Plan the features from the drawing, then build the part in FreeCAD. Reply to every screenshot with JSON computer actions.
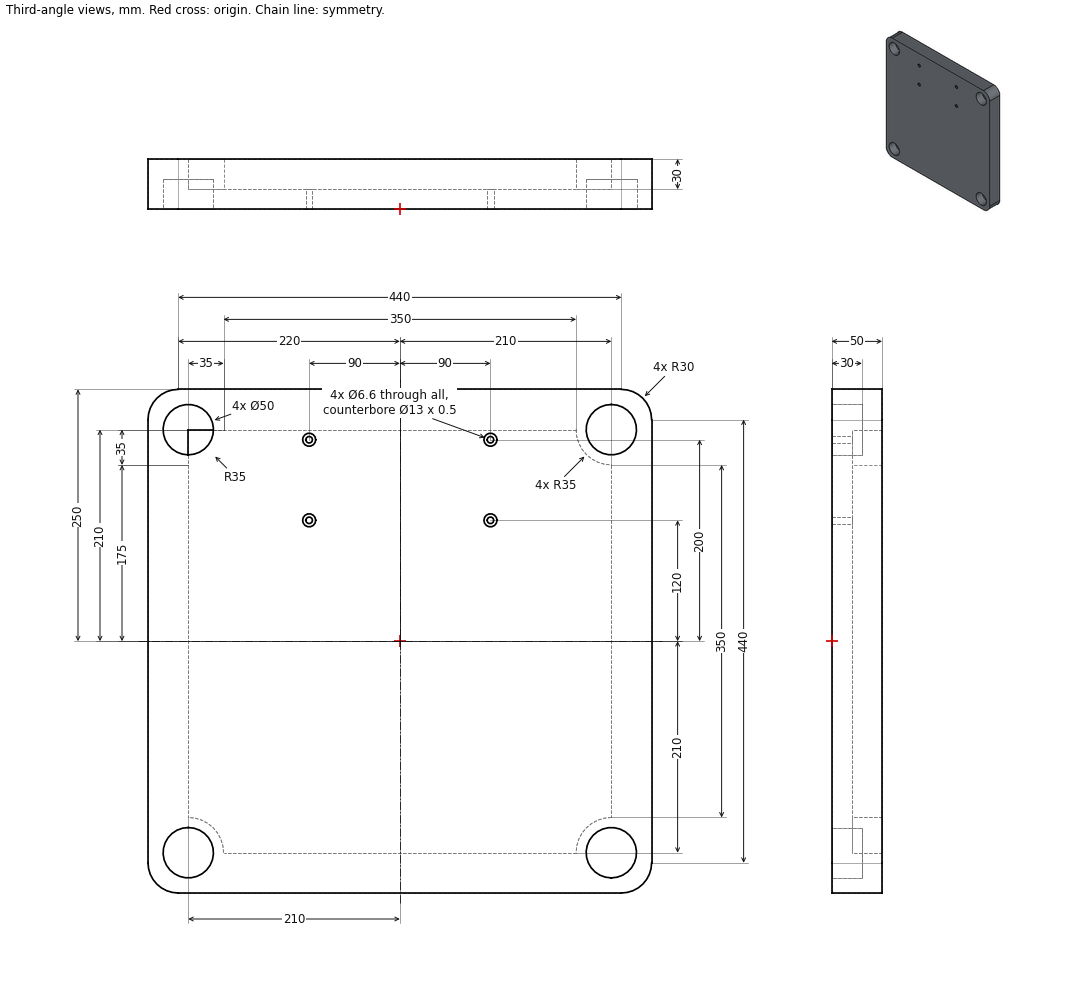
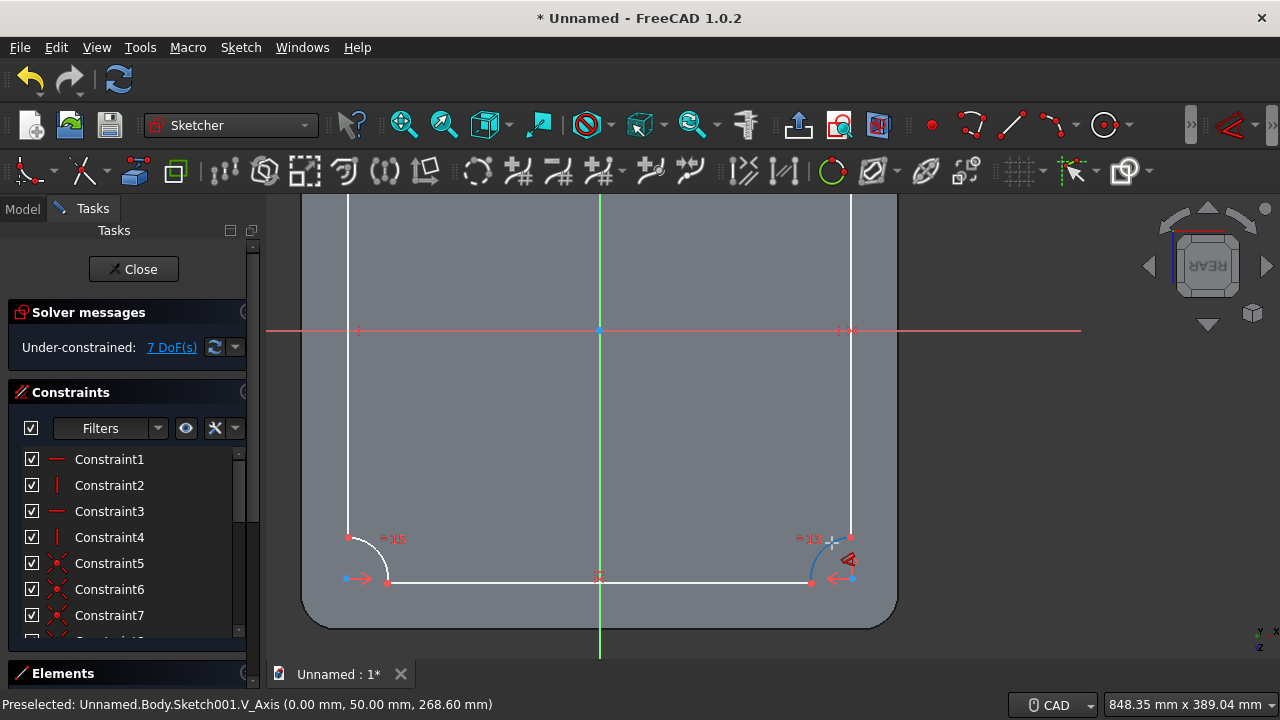
{"action": "left_click", "coordinate": [832, 543]}
{"action": "left_click", "coordinate": [816, 515]}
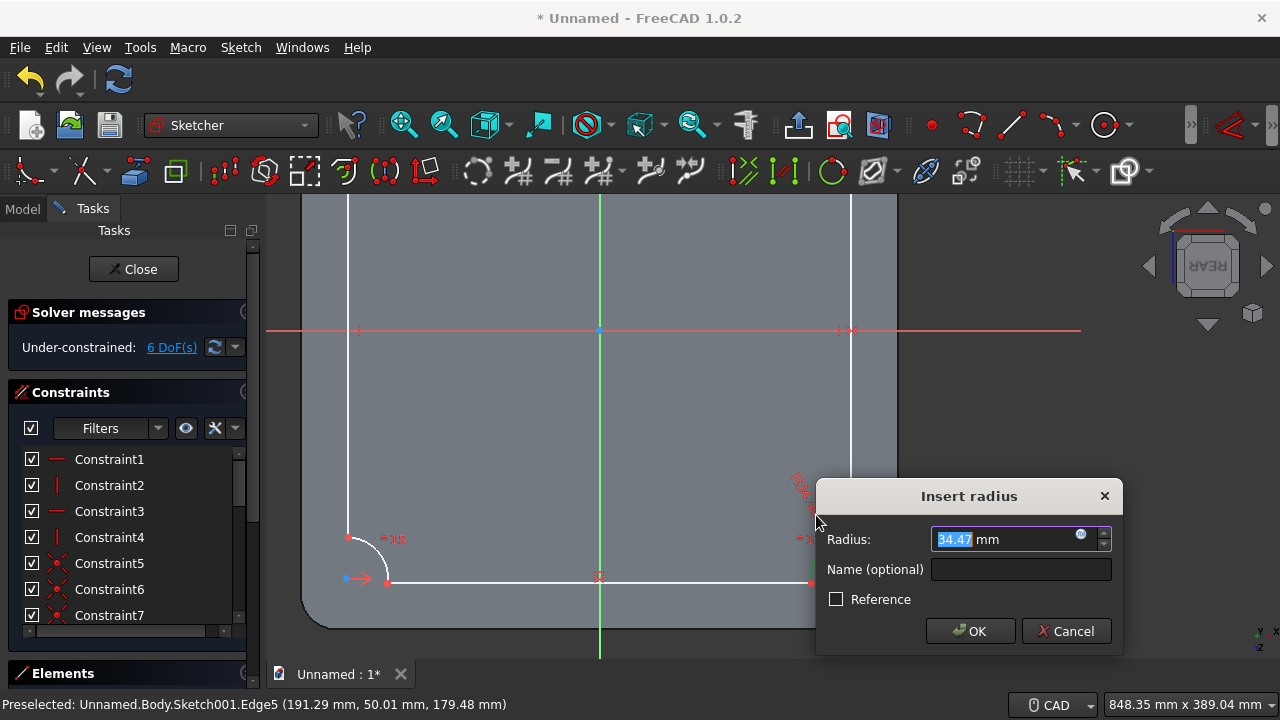
{"action": "type", "text": "35"}
{"action": "key", "text": "Return"}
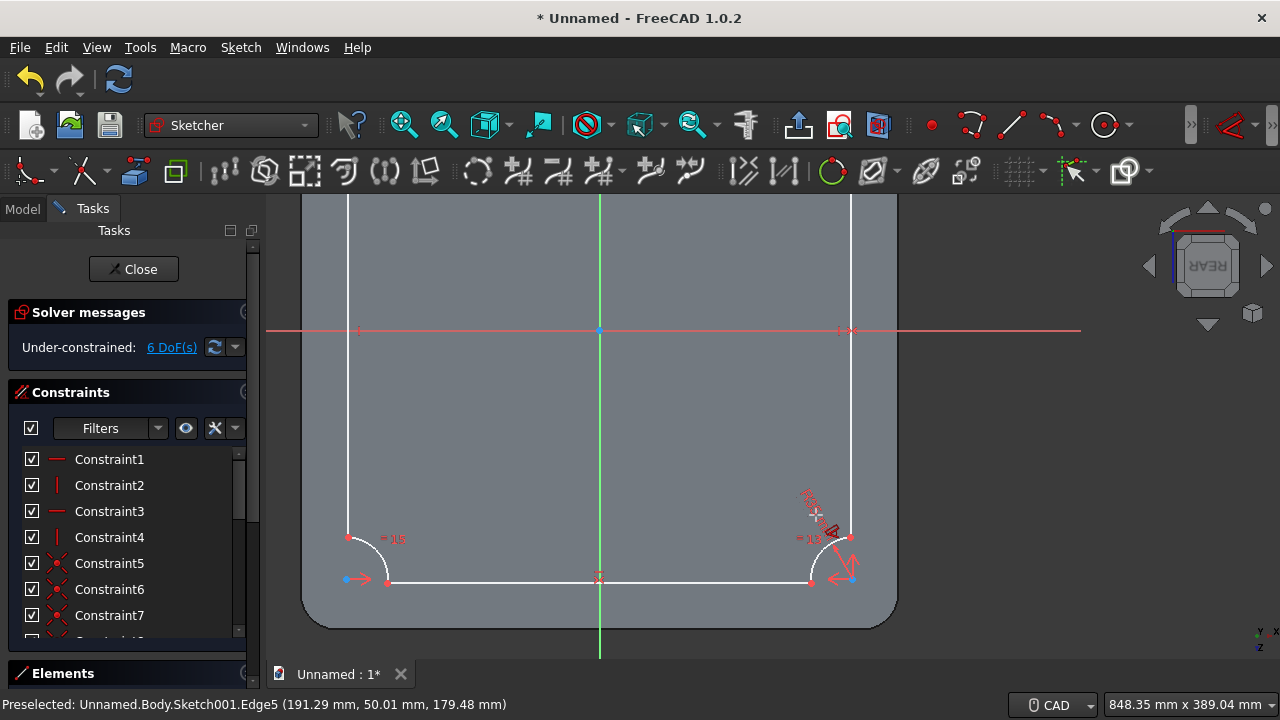
{"action": "left_click", "coordinate": [515, 583]}
{"action": "left_click", "coordinate": [502, 617]}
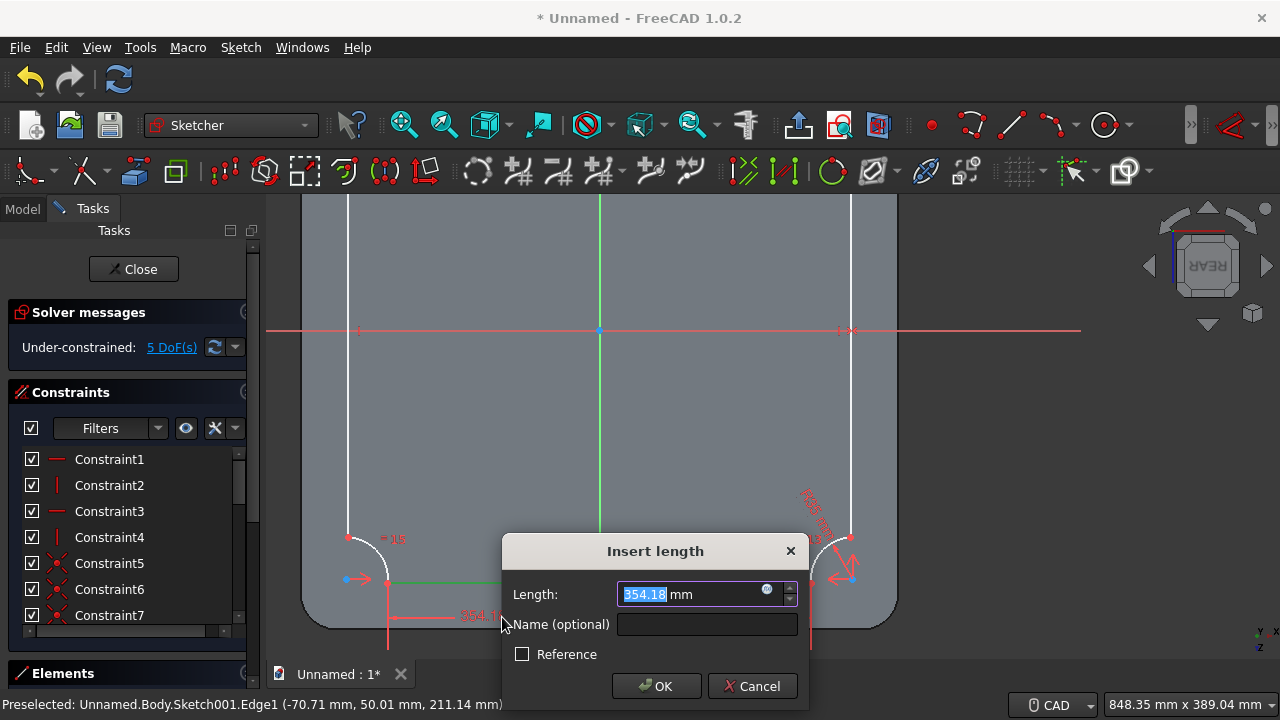
{"action": "type", "text": "350"}
{"action": "key", "text": "Return"}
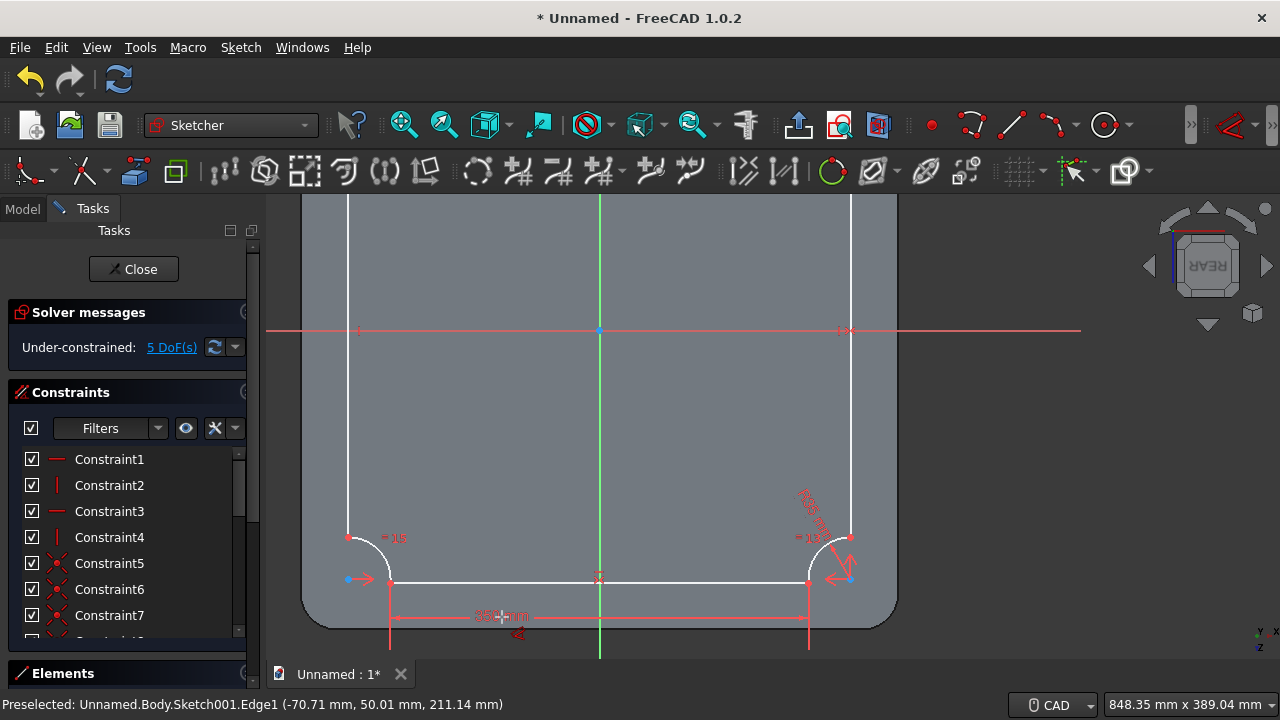
{"action": "left_click", "coordinate": [851, 413]}
{"action": "left_click", "coordinate": [885, 380]}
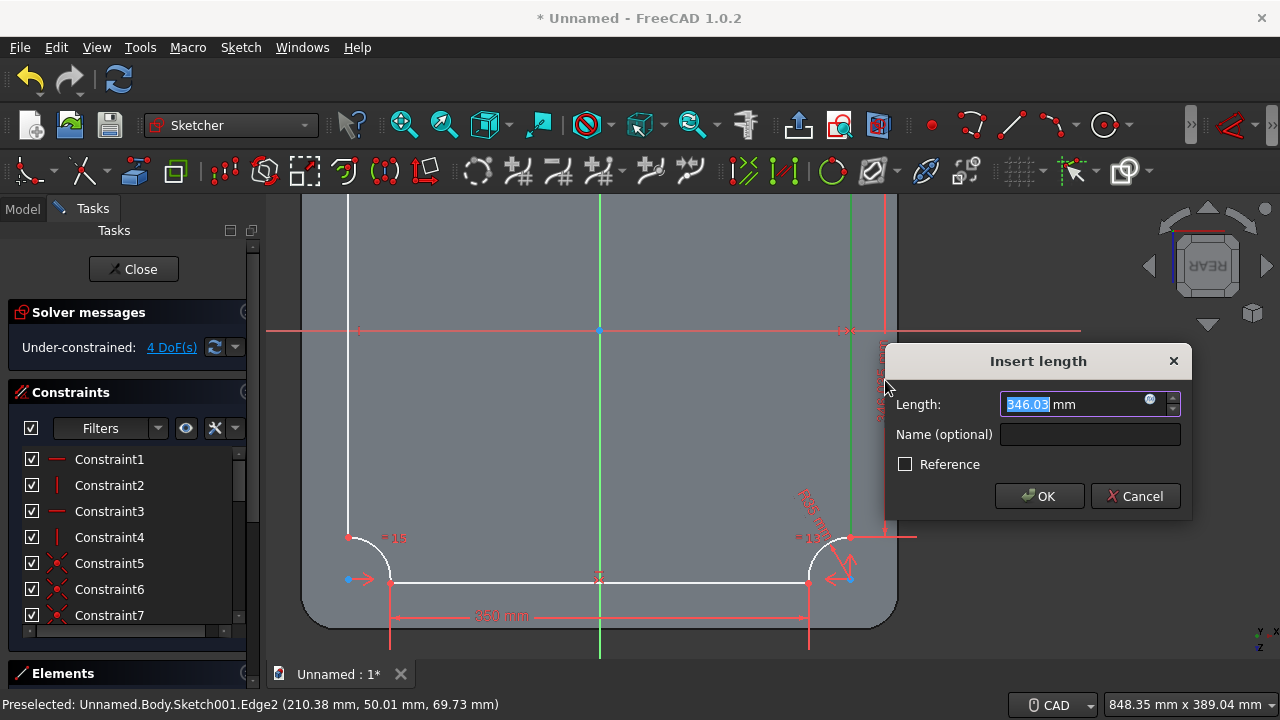
{"action": "type", "text": "350"}
{"action": "key", "text": "Return"}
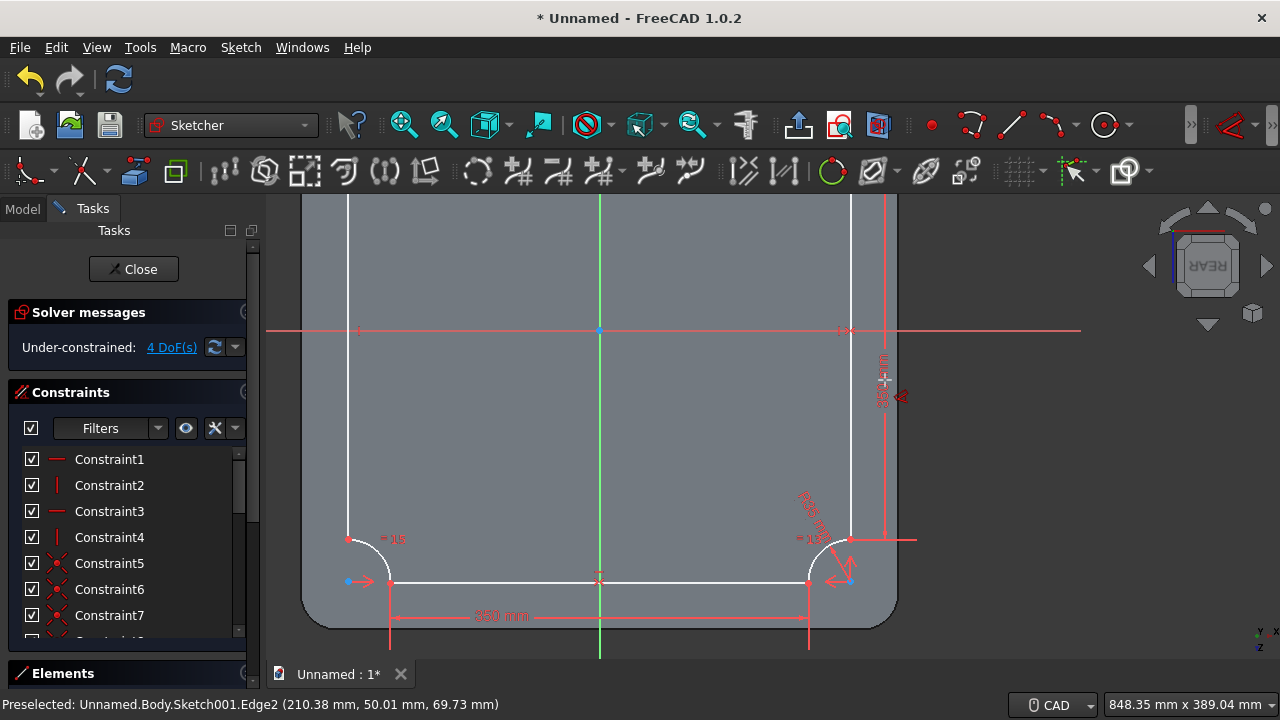
{"action": "left_click", "coordinate": [390, 583]}
{"action": "left_click", "coordinate": [634, 457]}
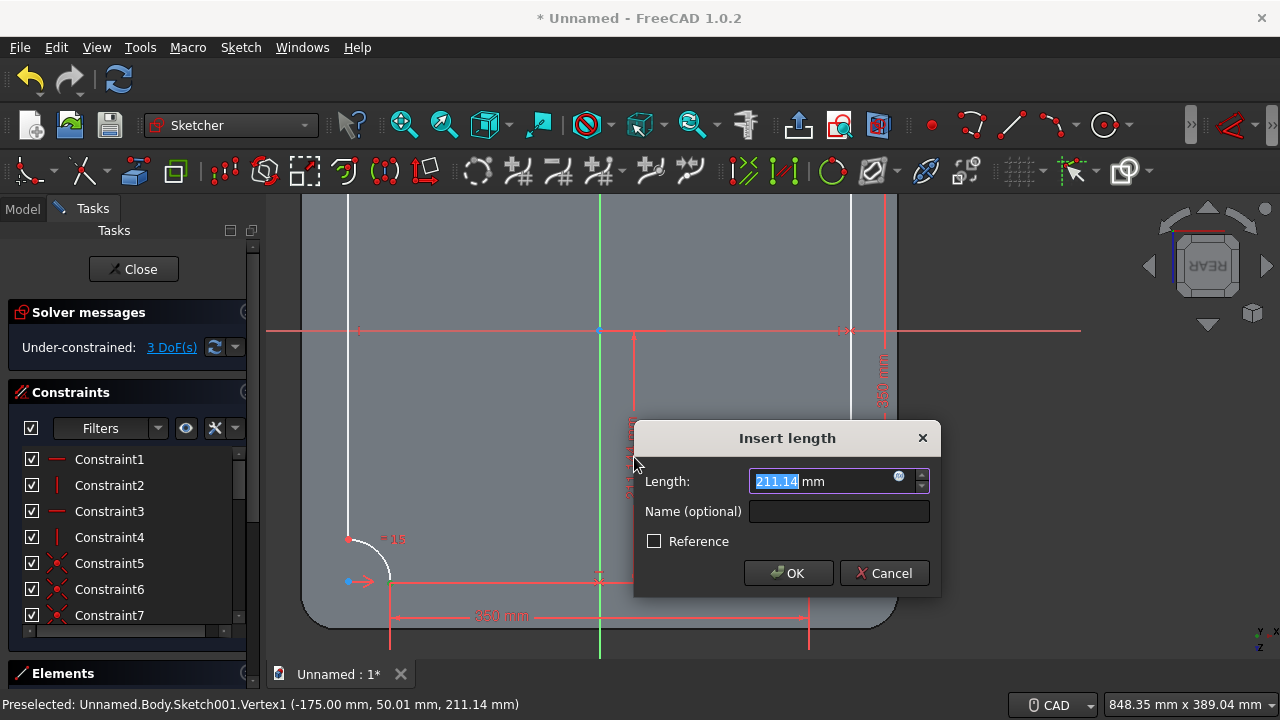
{"action": "type", "text": "210"}
{"action": "key", "text": "Return"}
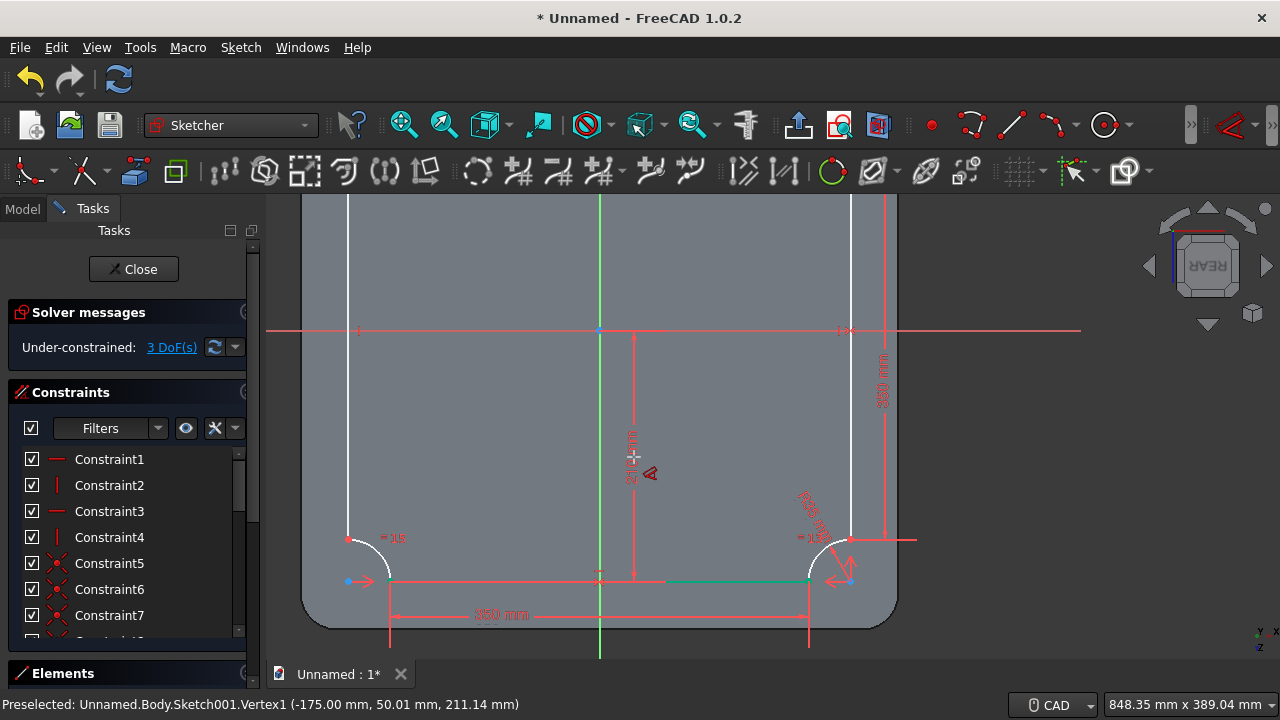
{"action": "left_click", "coordinate": [851, 540]}
{"action": "left_click", "coordinate": [725, 297]}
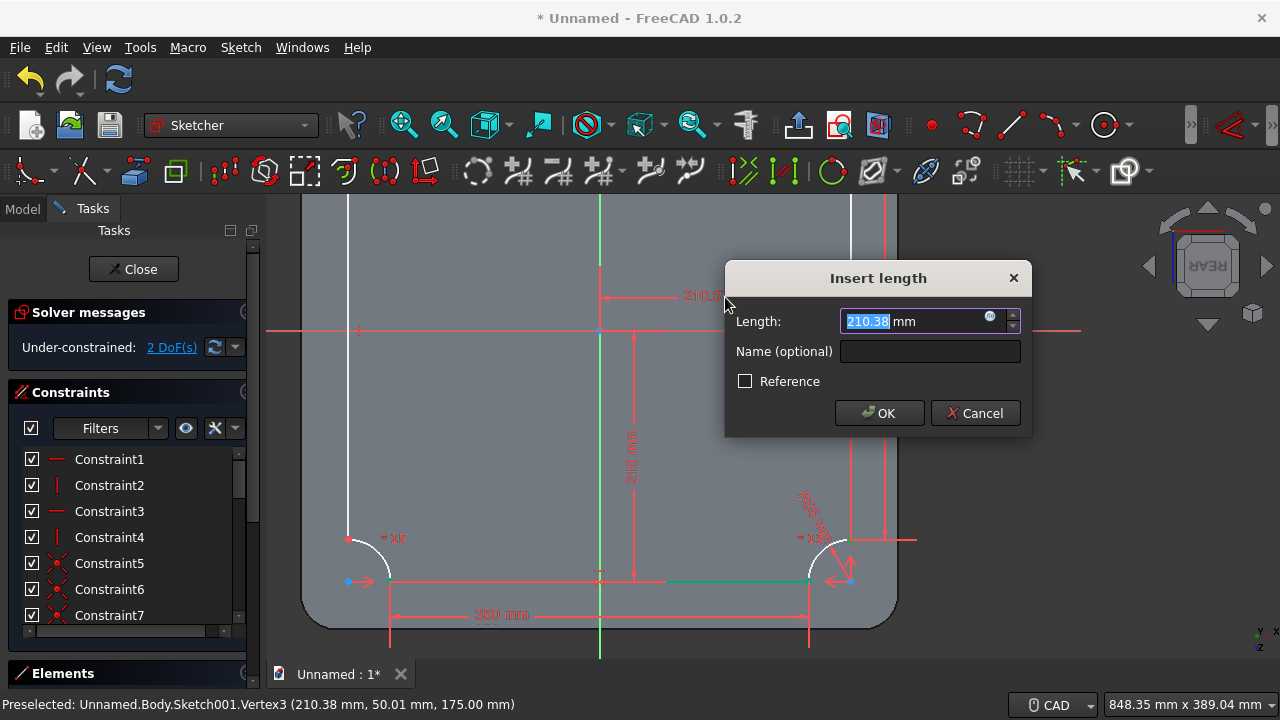
{"action": "type", "text": "210"}
{"action": "key", "text": "Return"}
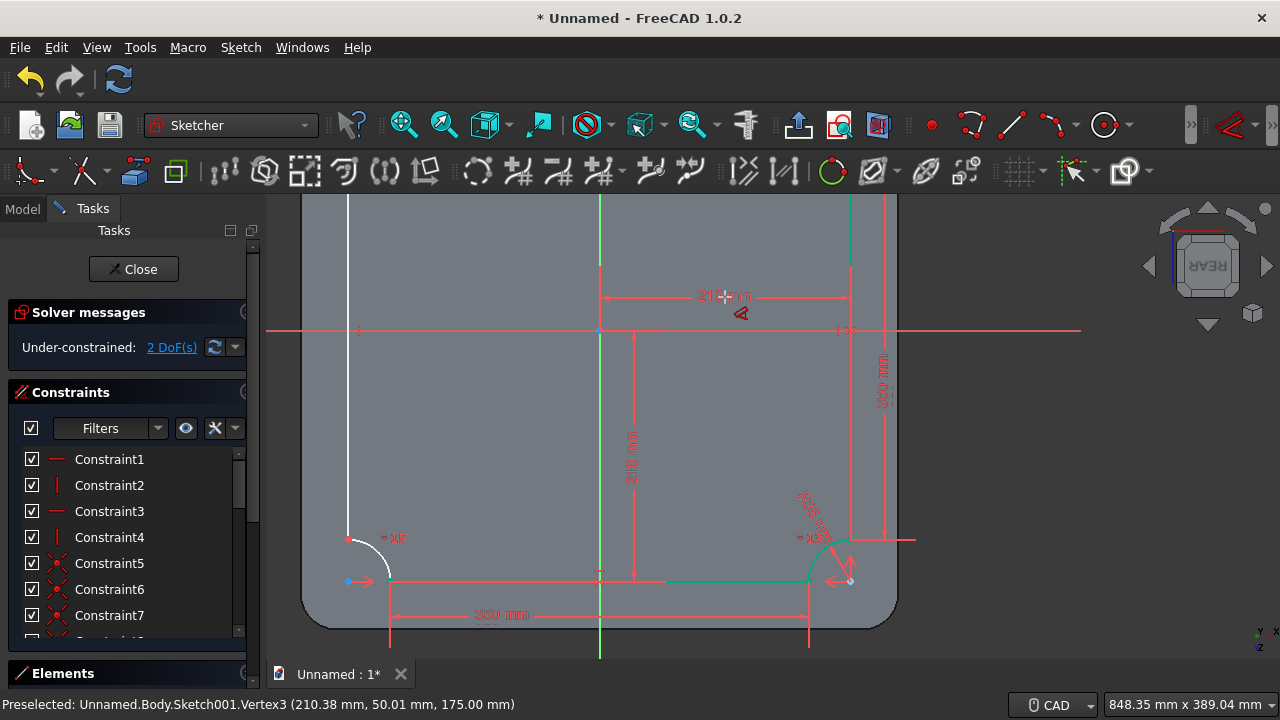
{"action": "scroll", "coordinate": [832, 543], "scroll_direction": "down", "scroll_amount": 3}